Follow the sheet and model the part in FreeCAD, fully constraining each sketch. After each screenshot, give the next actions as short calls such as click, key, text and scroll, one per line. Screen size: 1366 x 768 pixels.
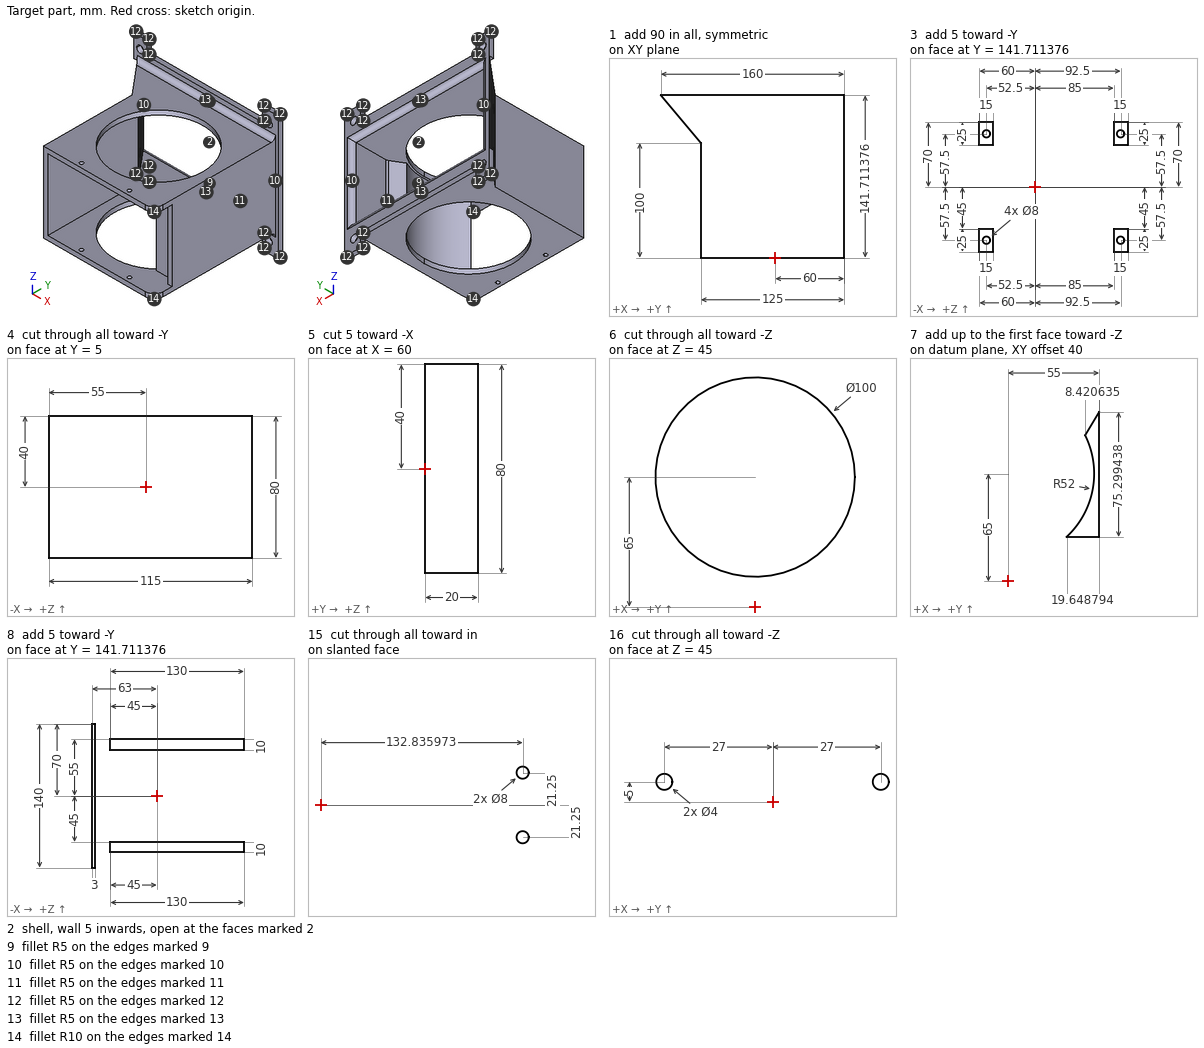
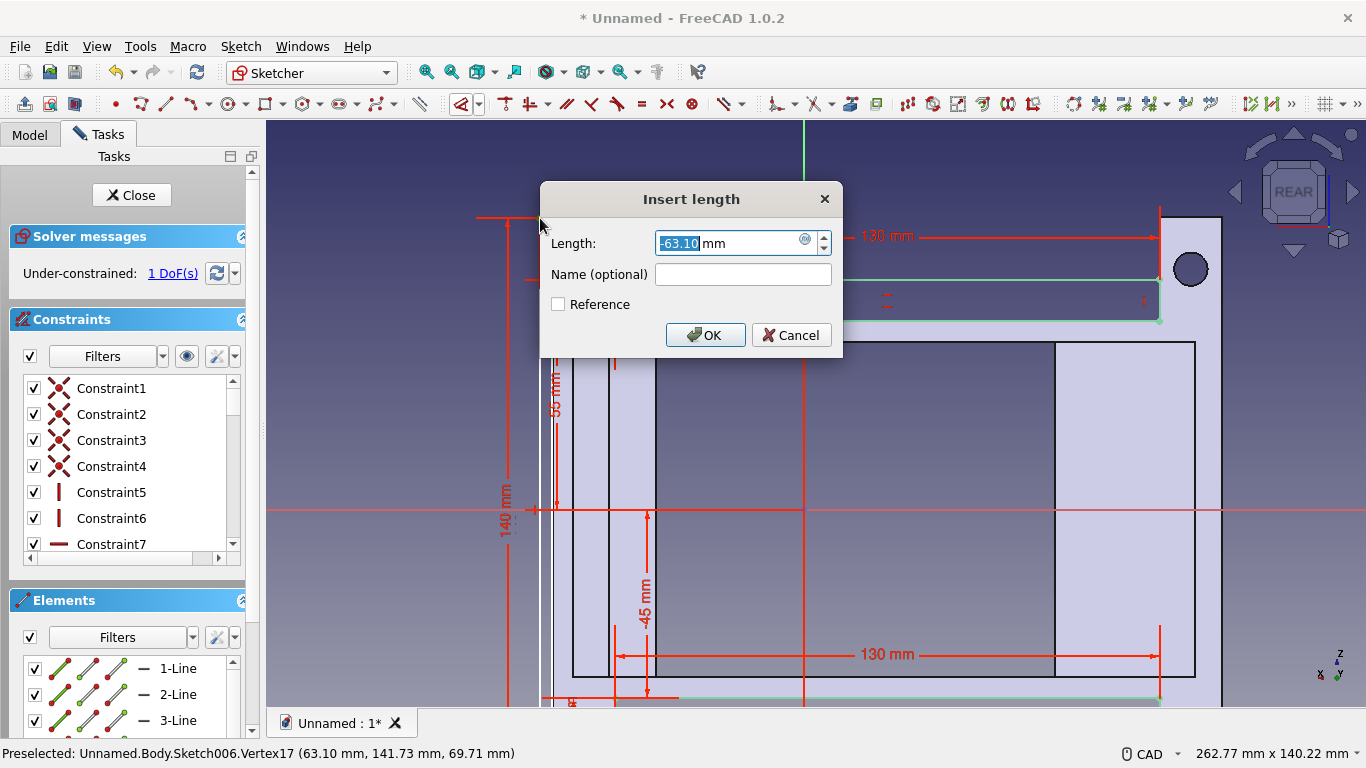
text(-63)
key(Return)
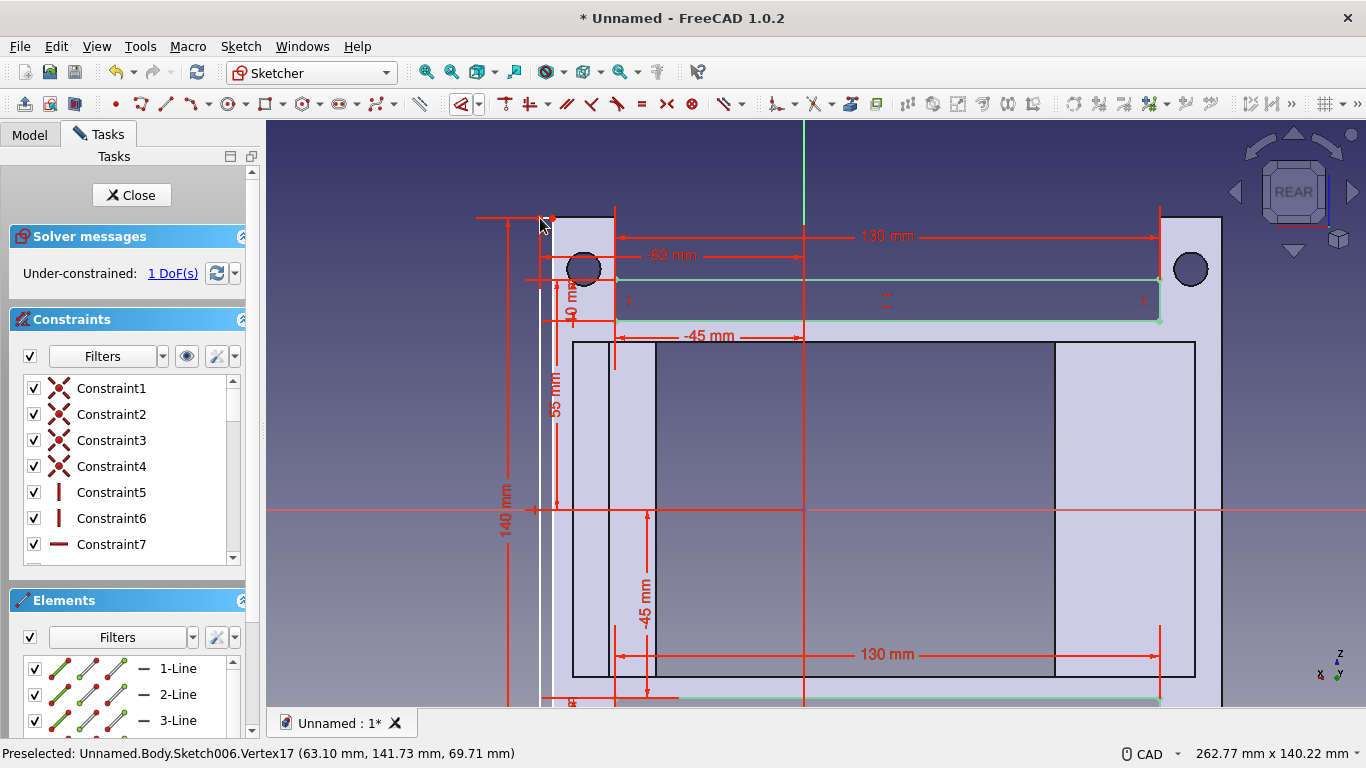
click(540, 218)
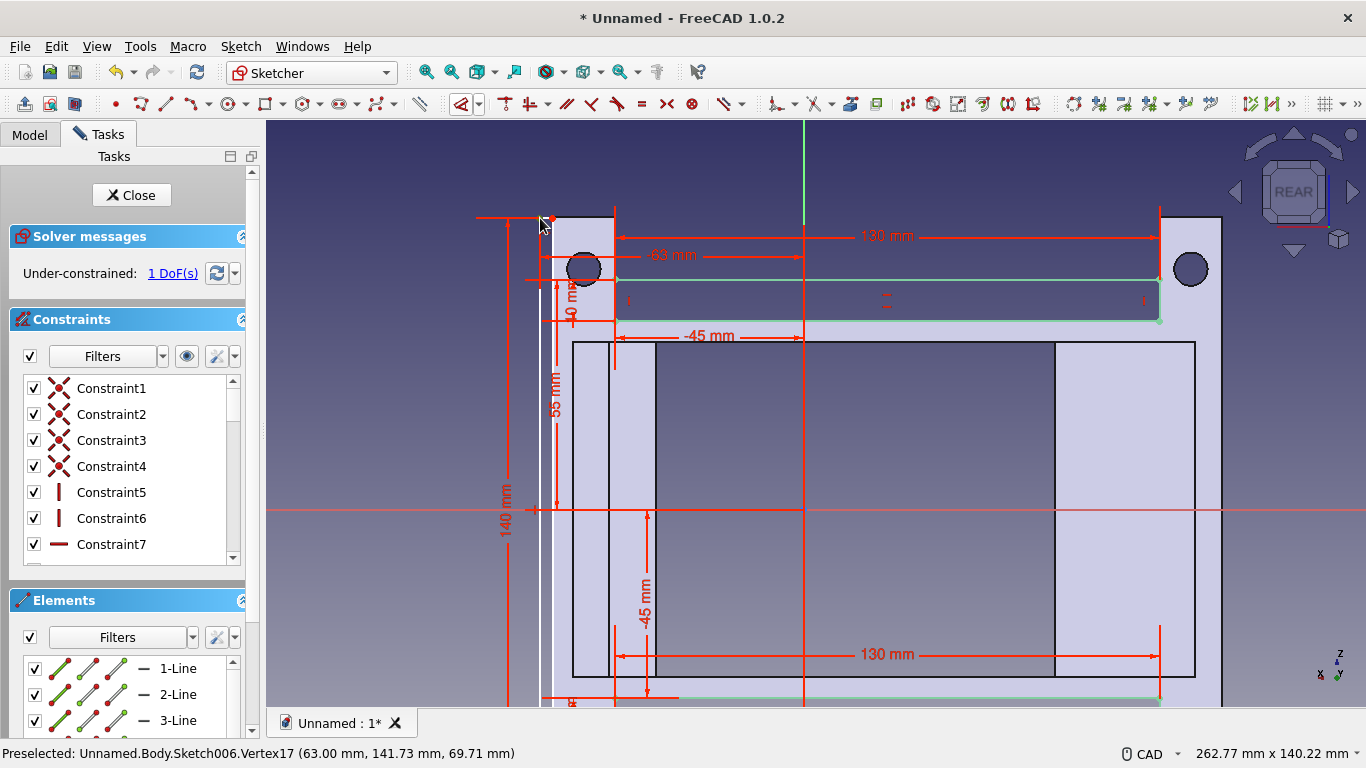
key(i)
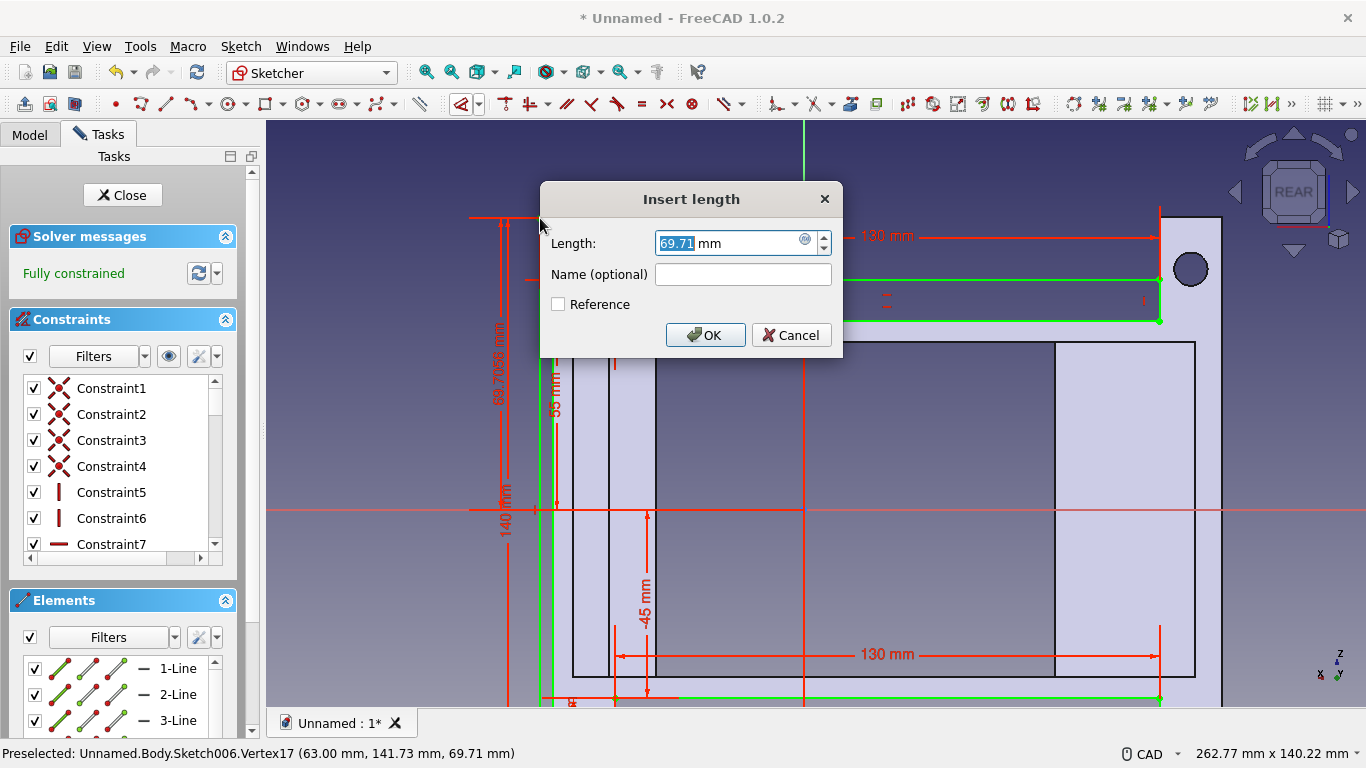
text(70)
key(Return)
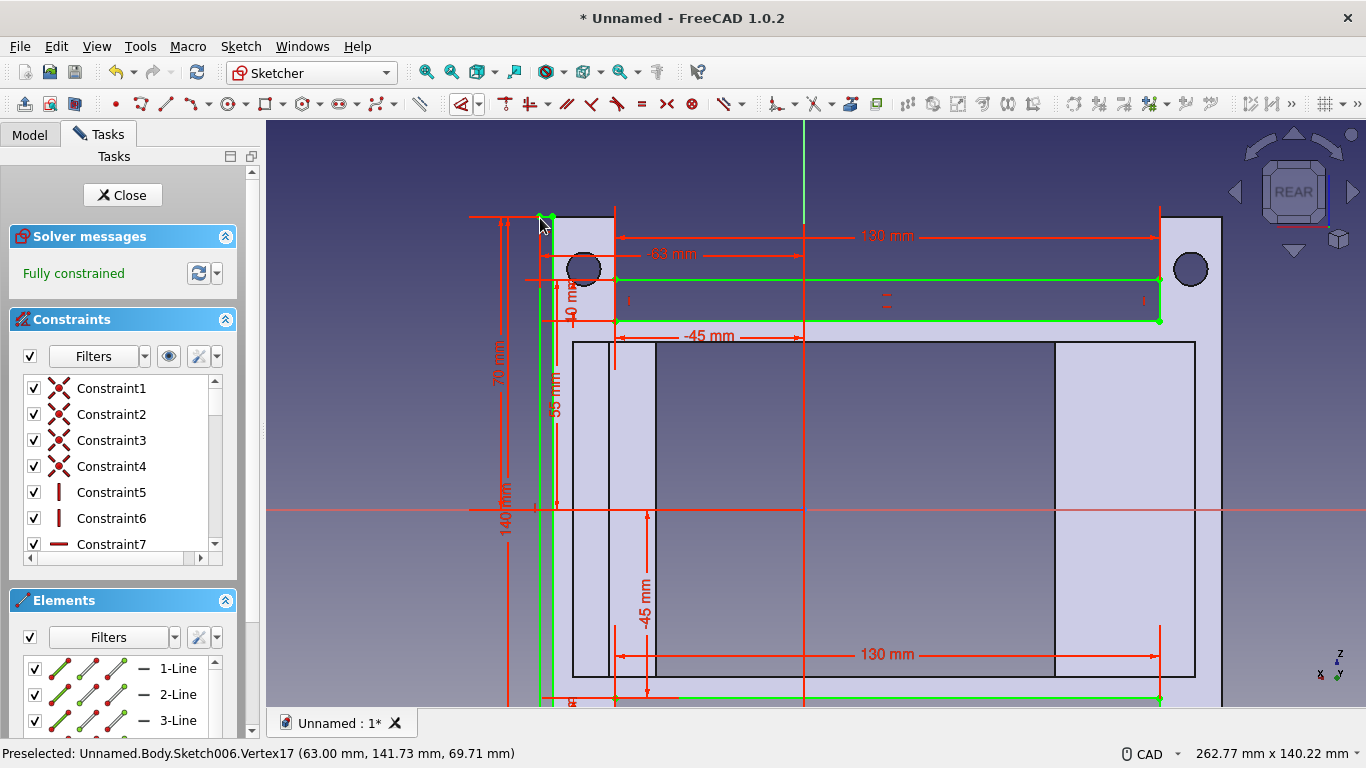
click(123, 195)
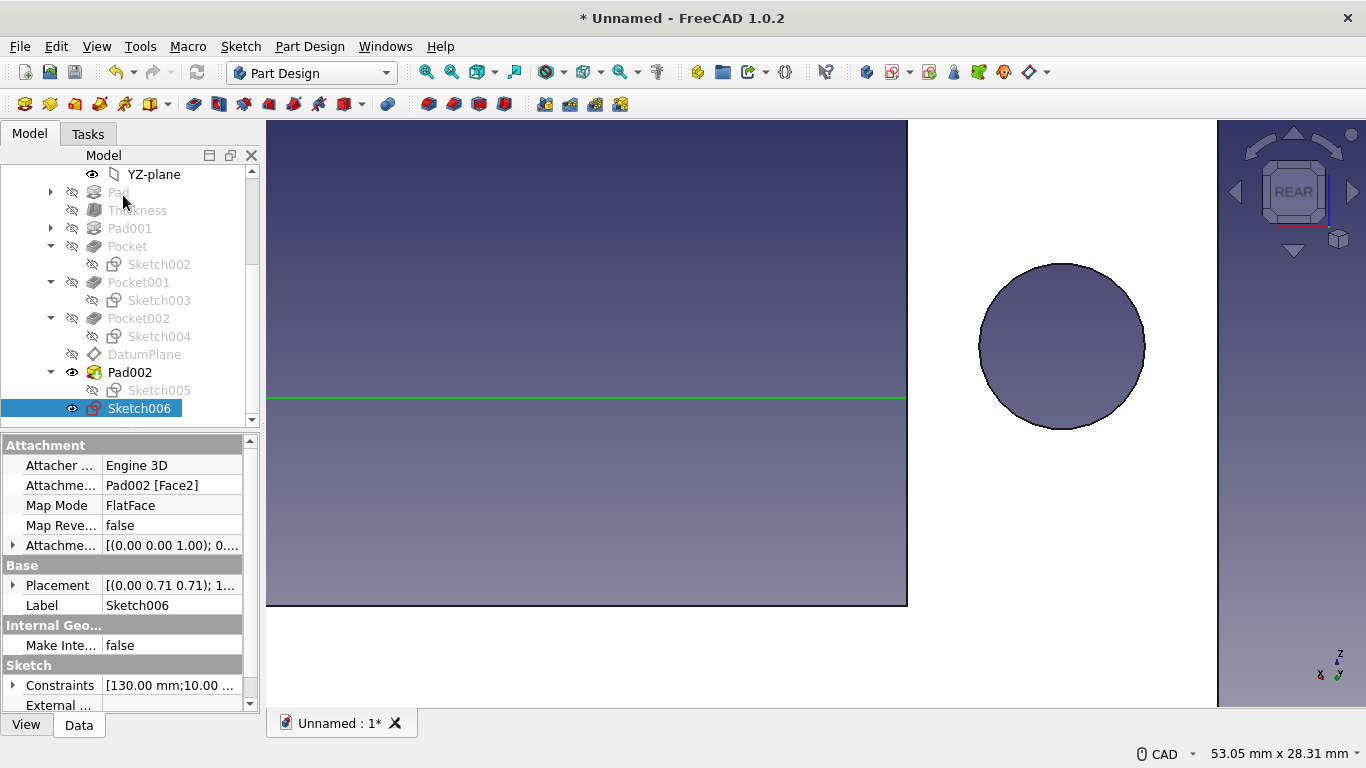
click(25, 104)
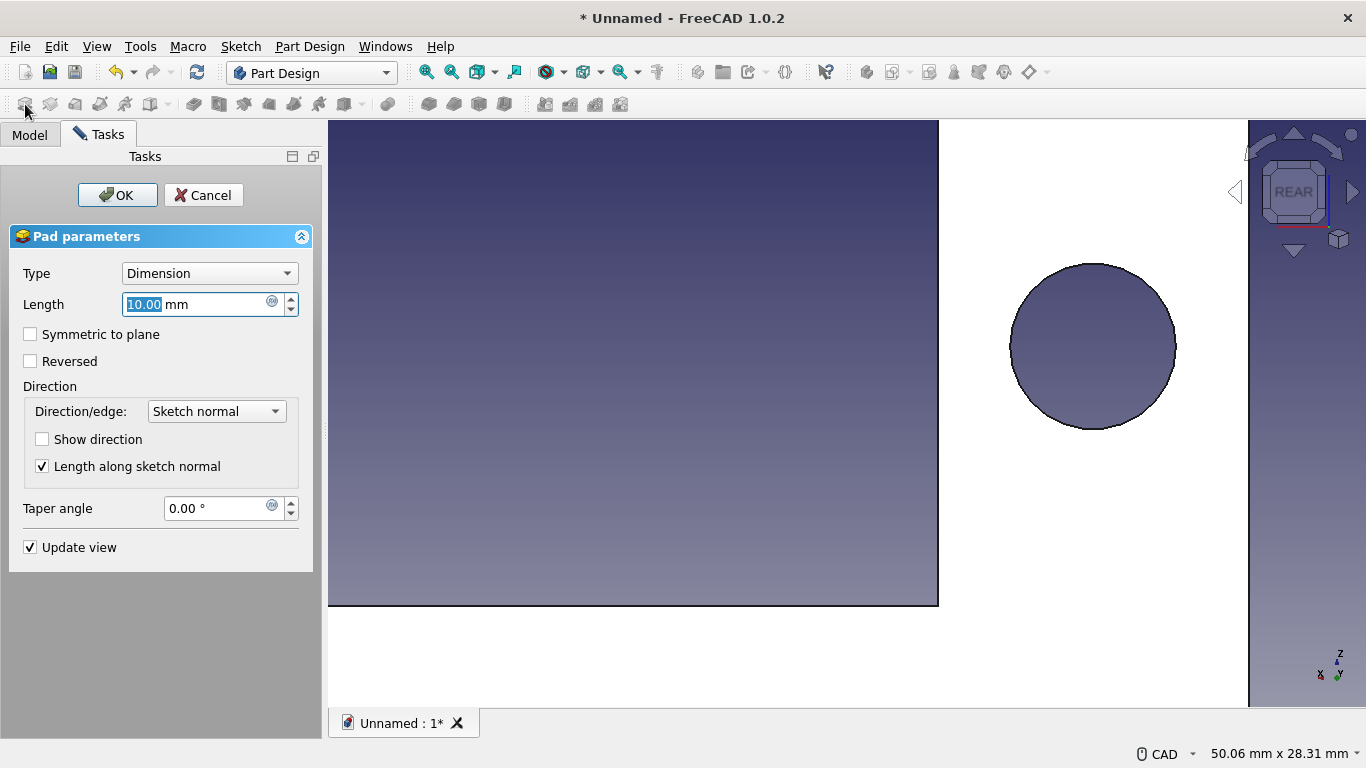
text(5)
key(Tab)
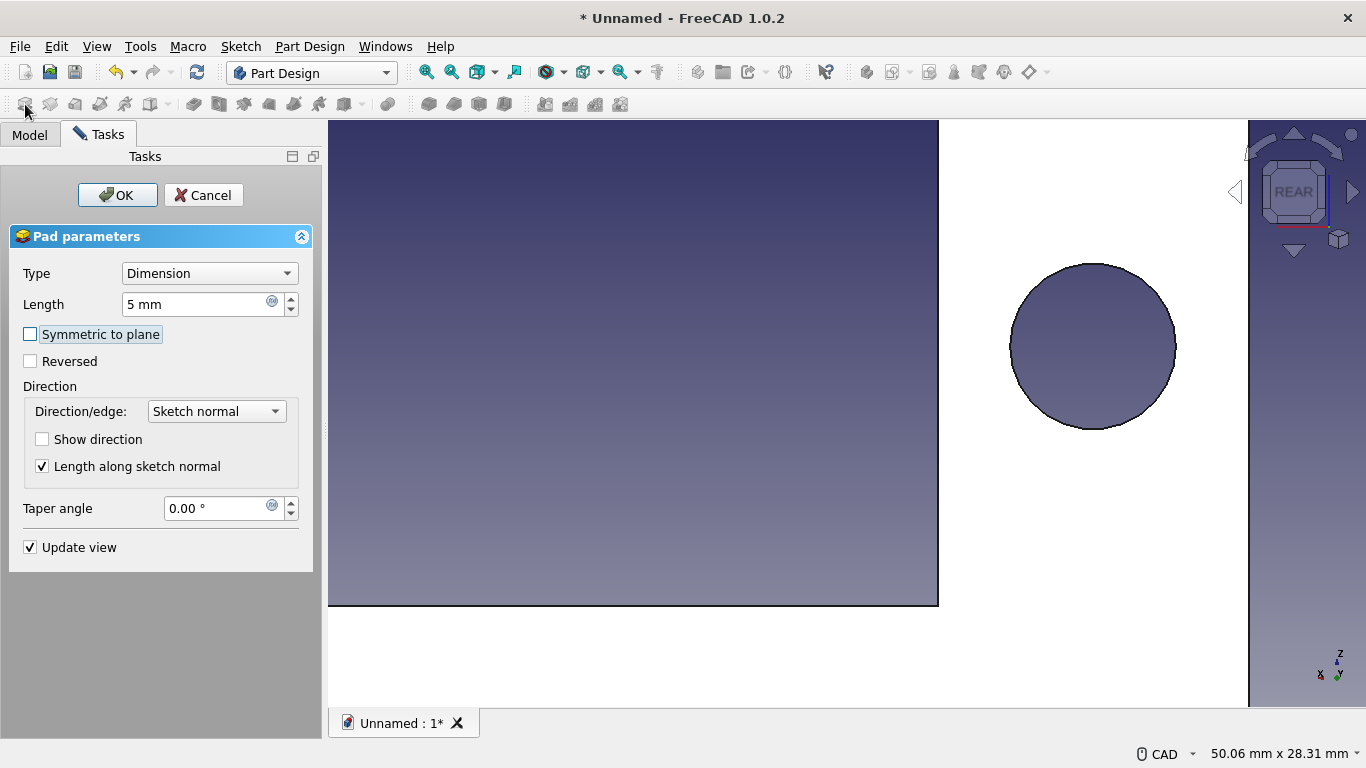
click(31, 361)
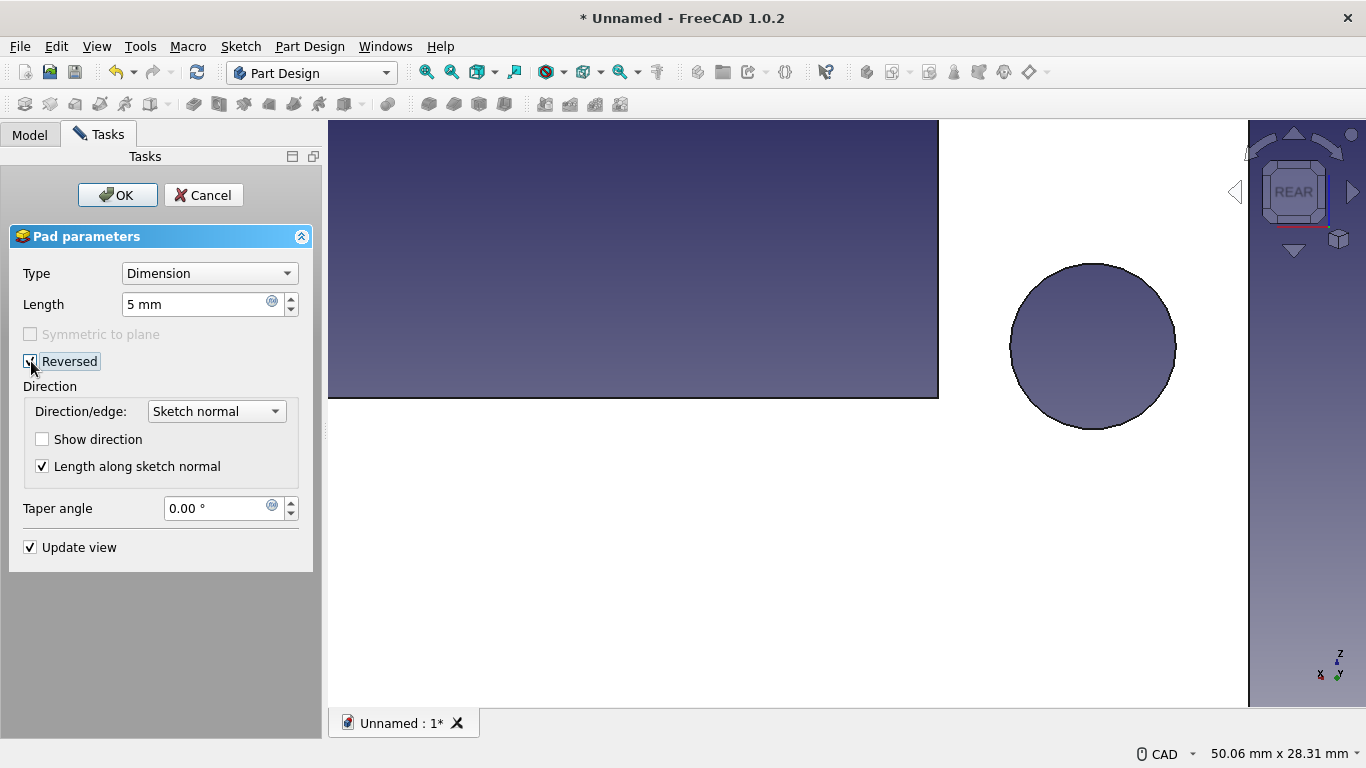
click(118, 195)